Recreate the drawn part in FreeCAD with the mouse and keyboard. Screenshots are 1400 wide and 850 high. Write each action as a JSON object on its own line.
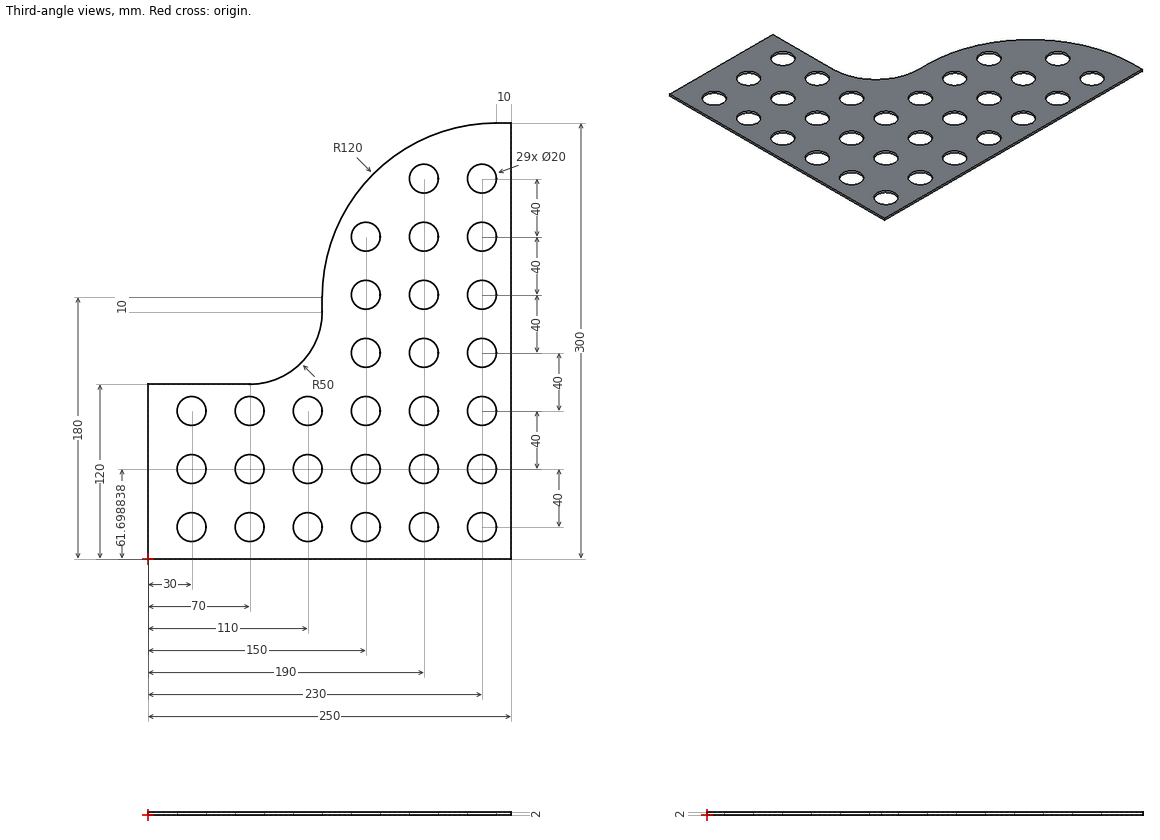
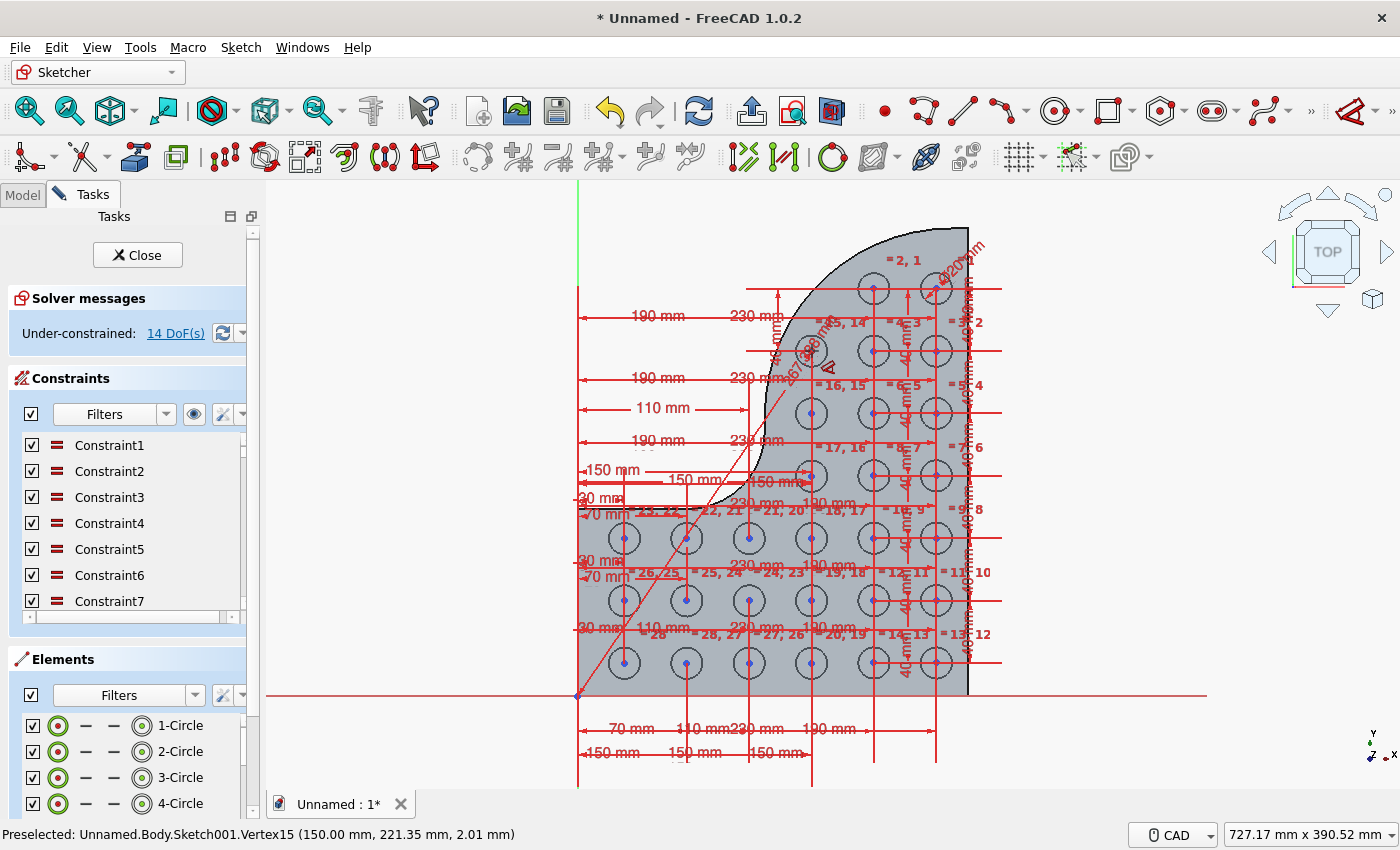
{"action": "left_click", "coordinate": [812, 414]}
{"action": "left_click", "coordinate": [846, 382]}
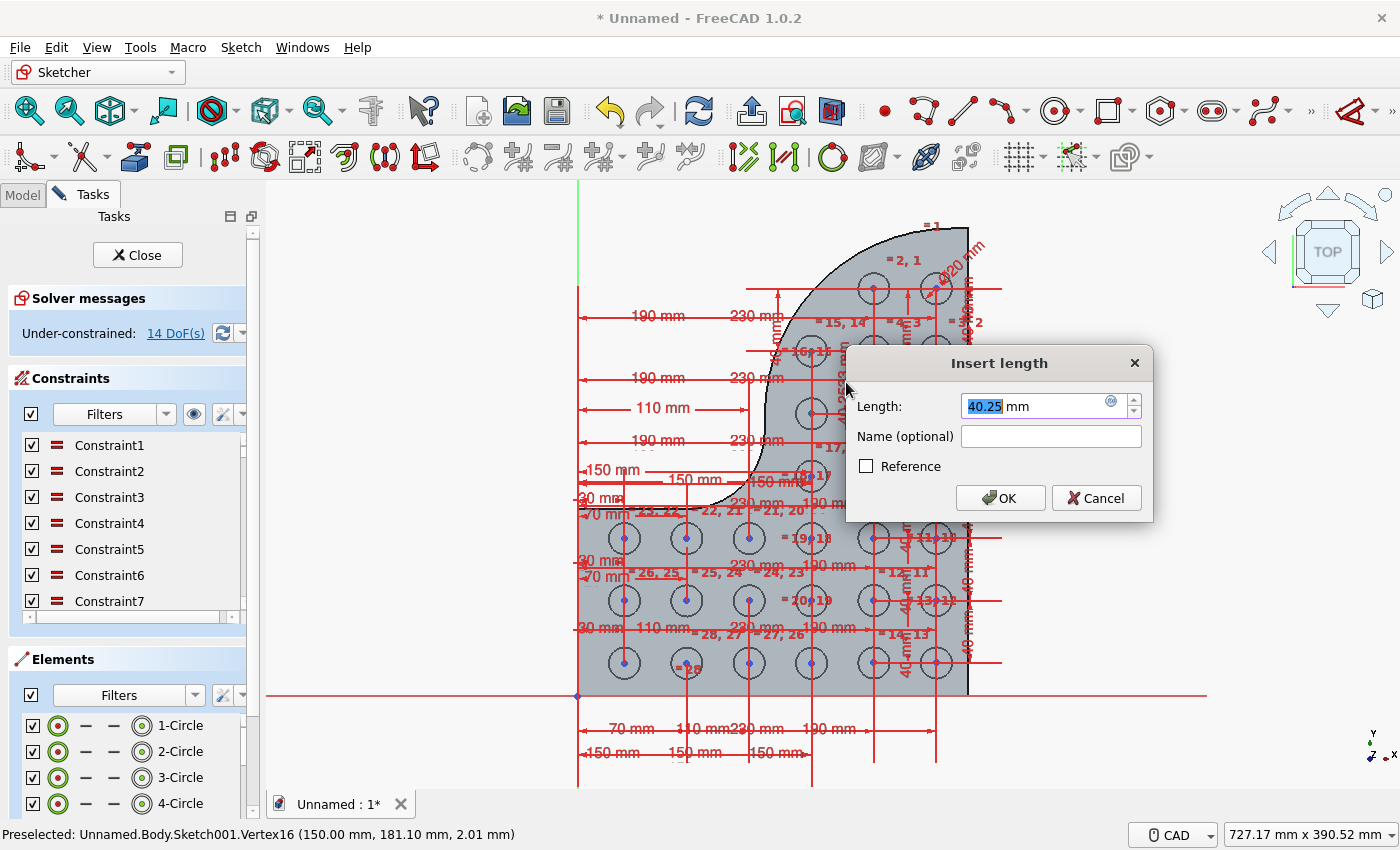
{"action": "type", "text": "40"}
{"action": "key", "text": "Return"}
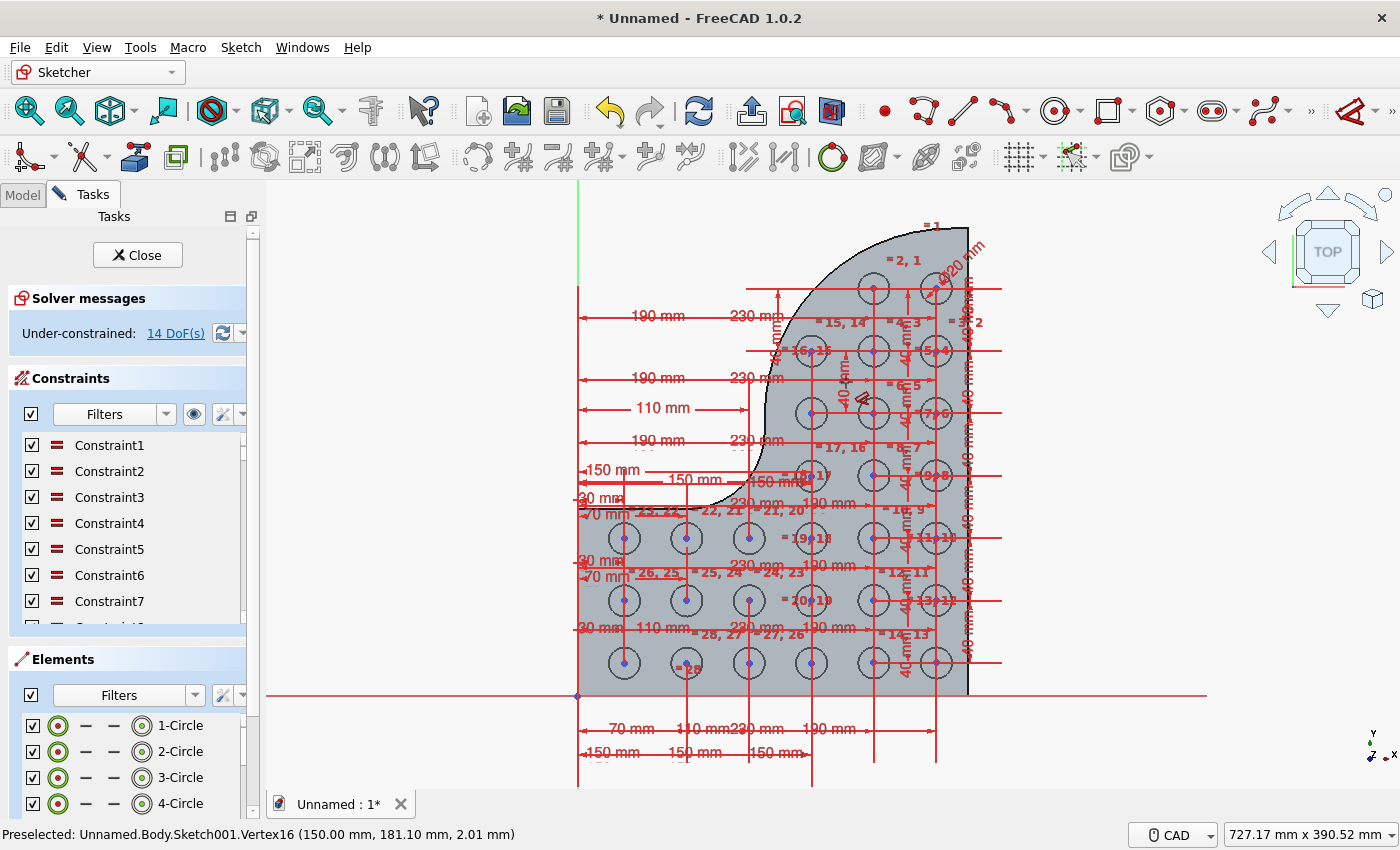
{"action": "left_click", "coordinate": [812, 413]}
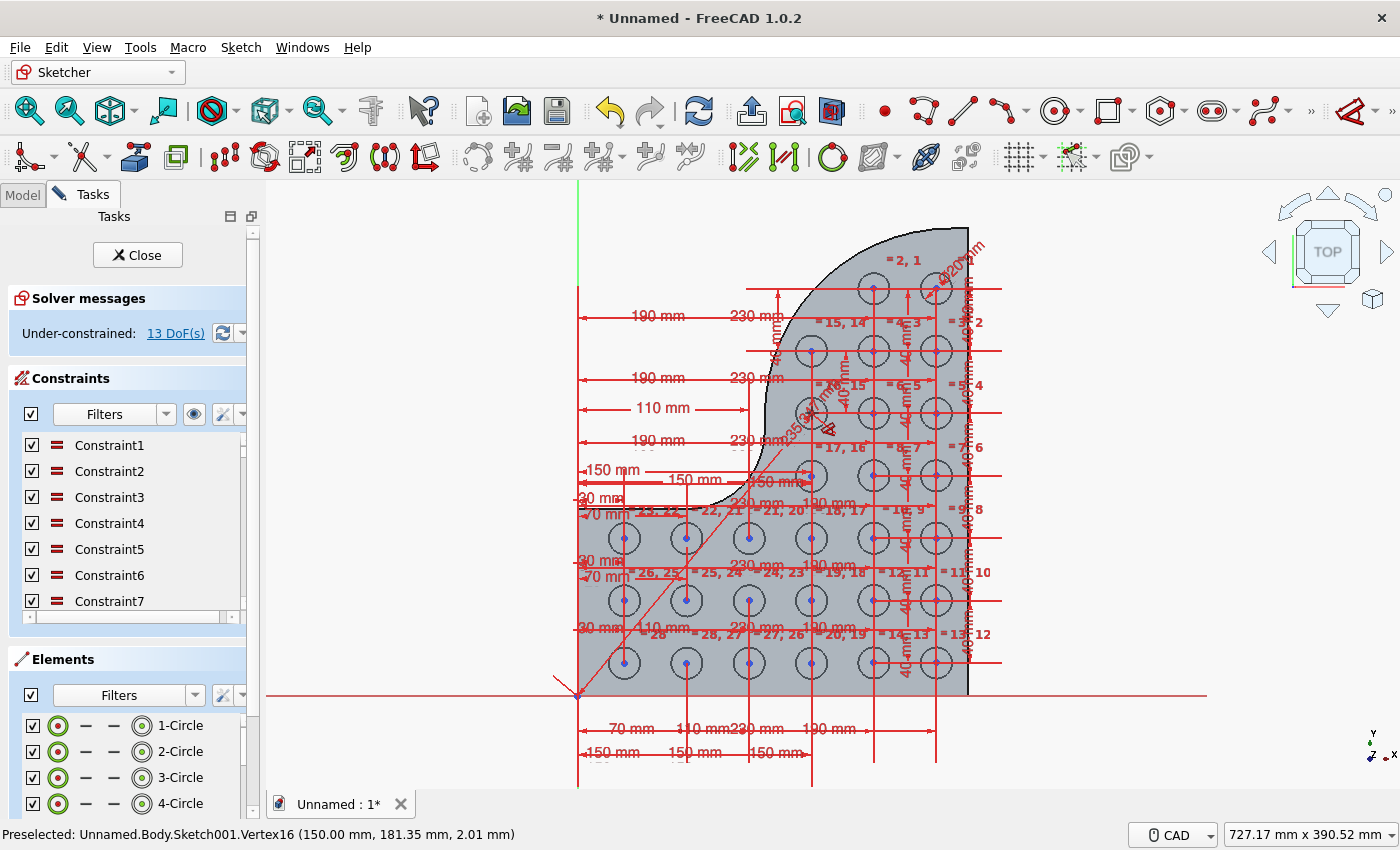
{"action": "left_click", "coordinate": [812, 476]}
{"action": "left_click", "coordinate": [846, 445]}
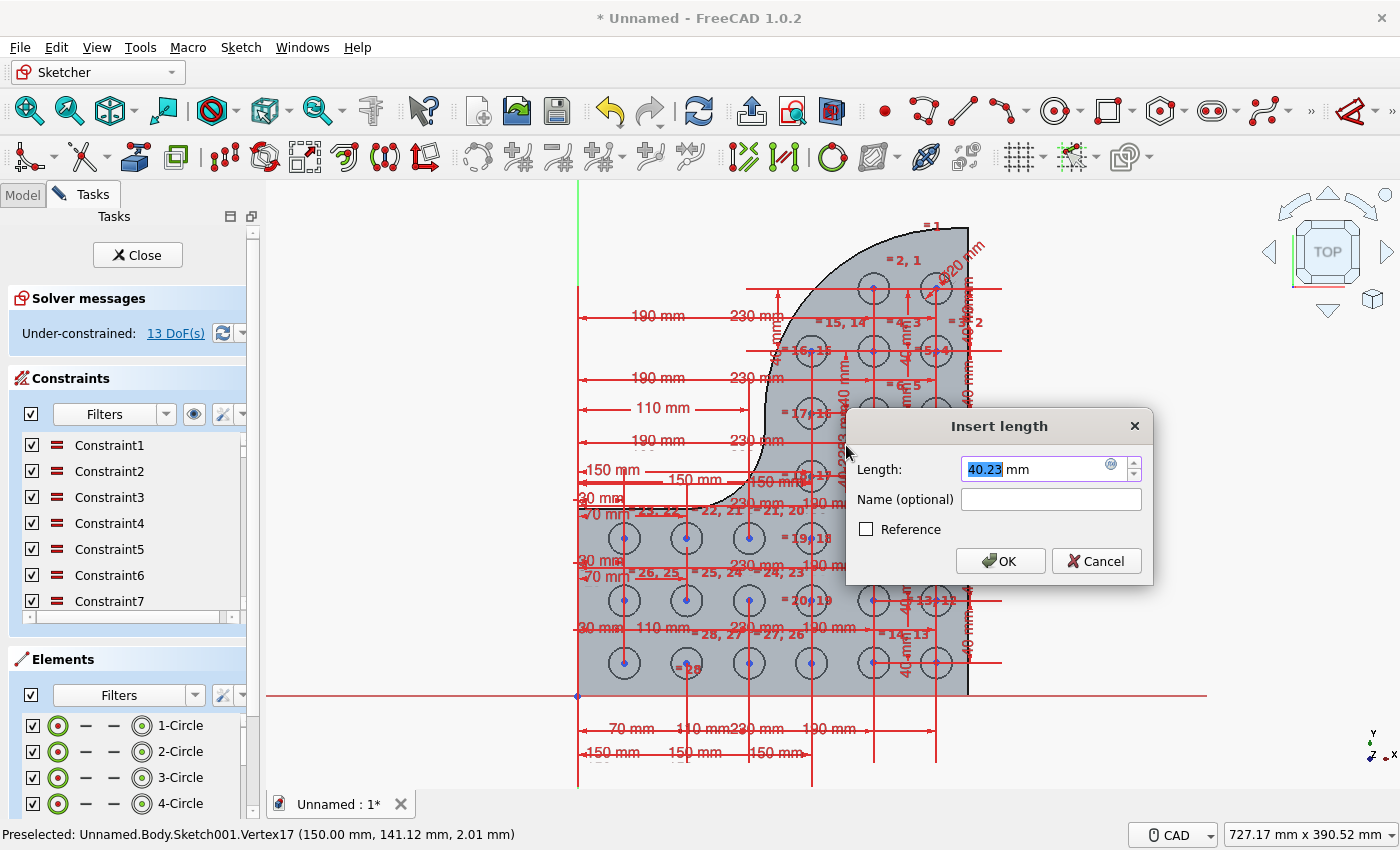
{"action": "type", "text": "40"}
{"action": "key", "text": "Return"}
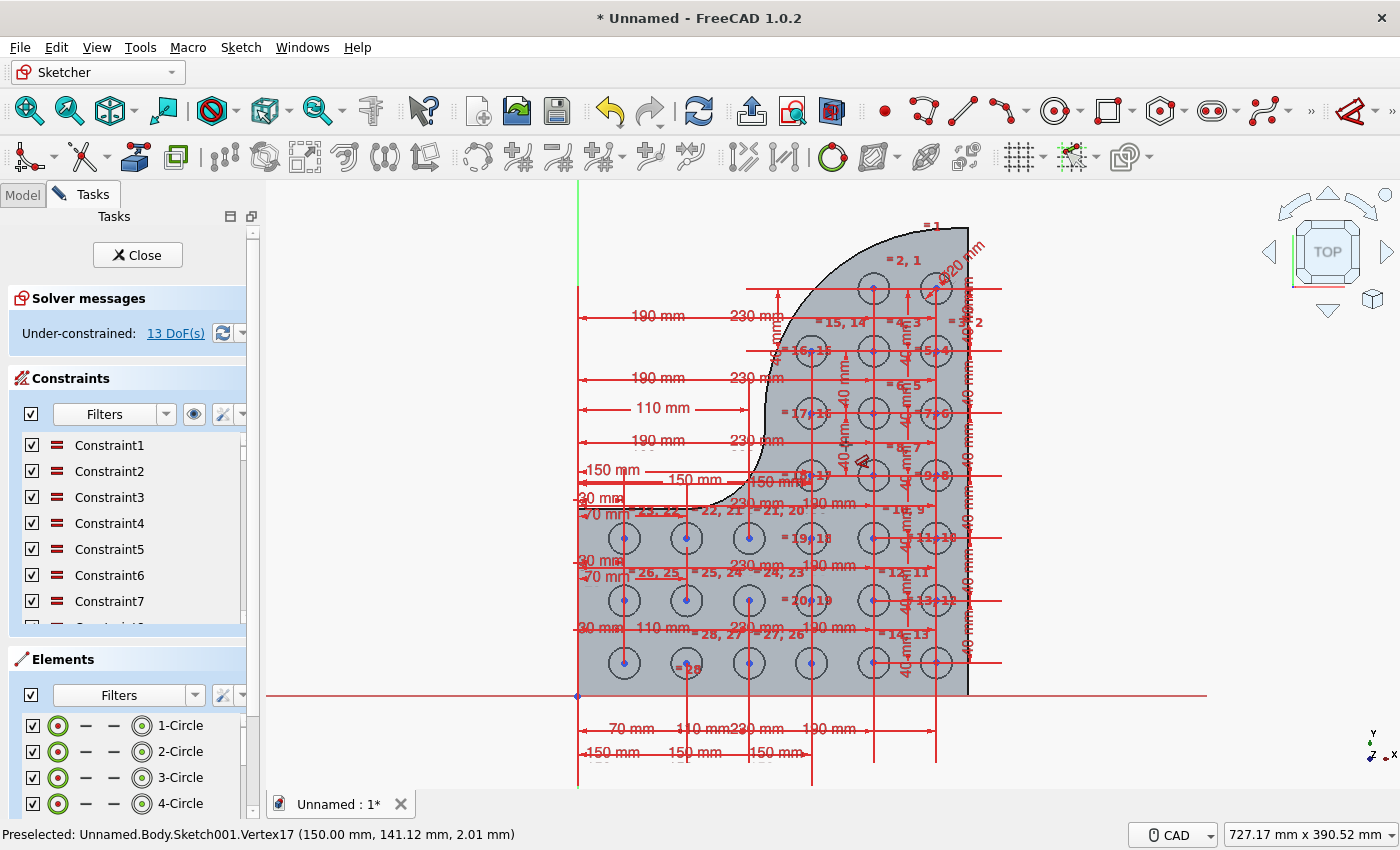
{"action": "left_click", "coordinate": [812, 476]}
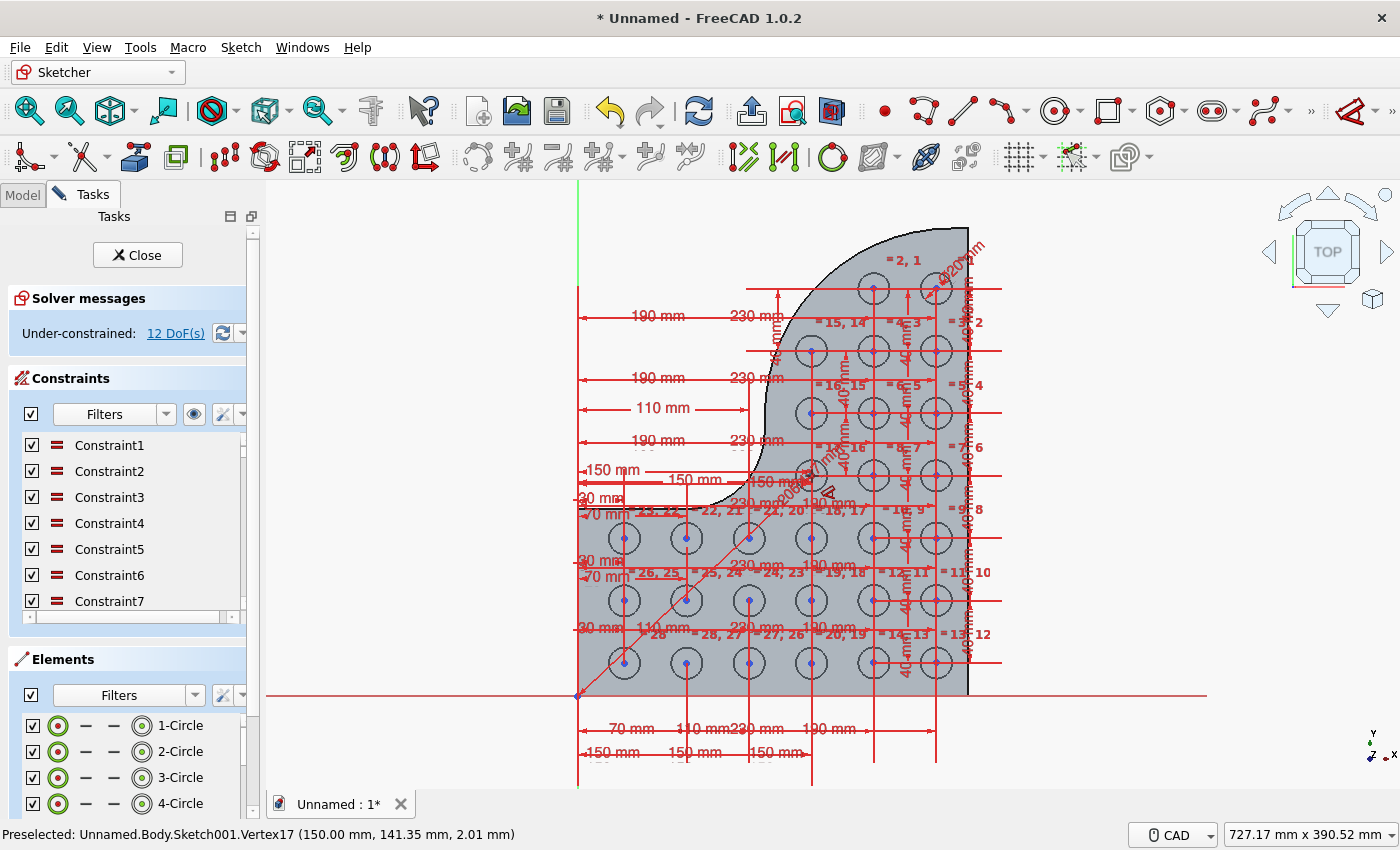
{"action": "left_click", "coordinate": [812, 539]}
{"action": "left_click", "coordinate": [778, 529]}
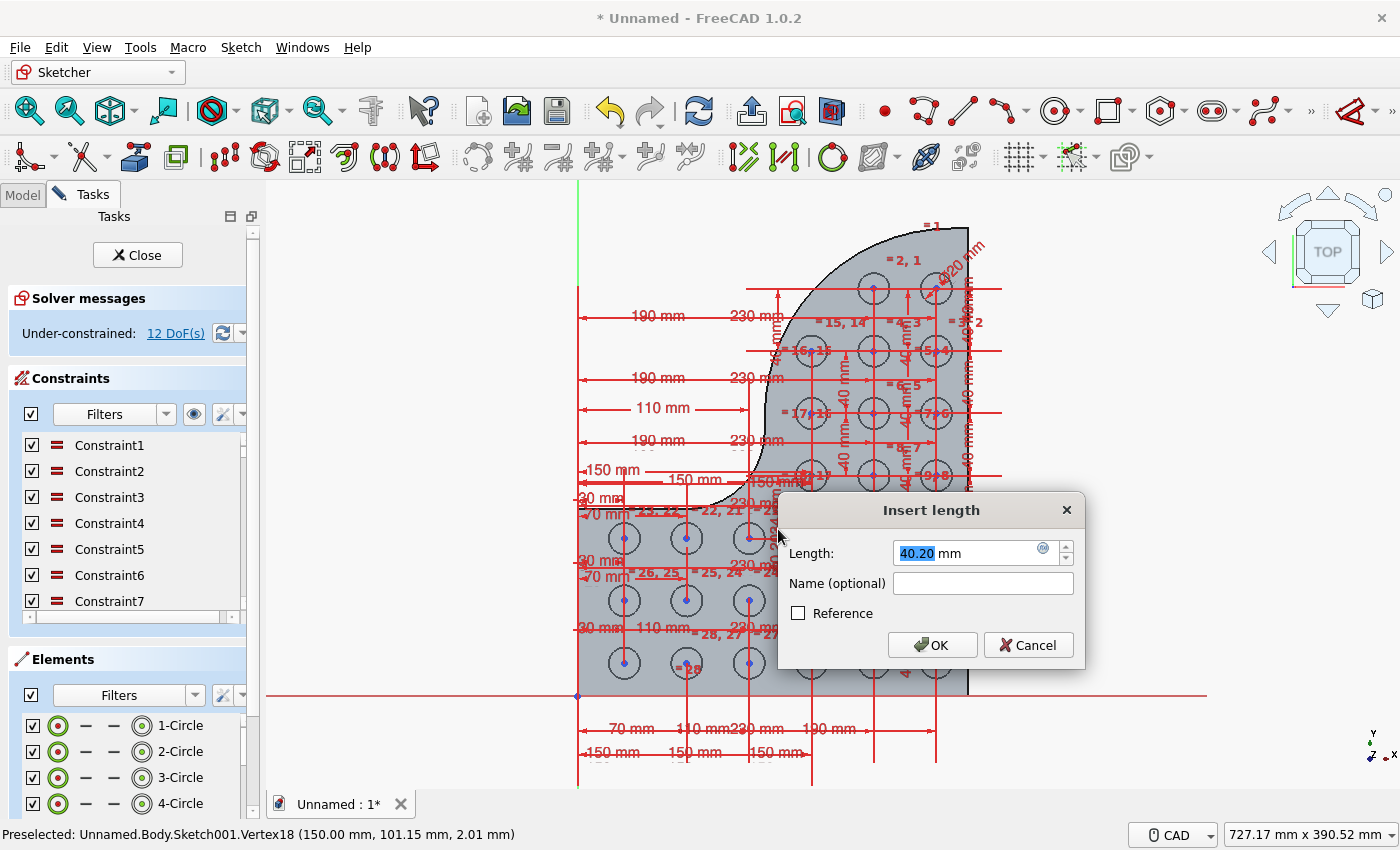
{"action": "type", "text": "40"}
{"action": "key", "text": "Return"}